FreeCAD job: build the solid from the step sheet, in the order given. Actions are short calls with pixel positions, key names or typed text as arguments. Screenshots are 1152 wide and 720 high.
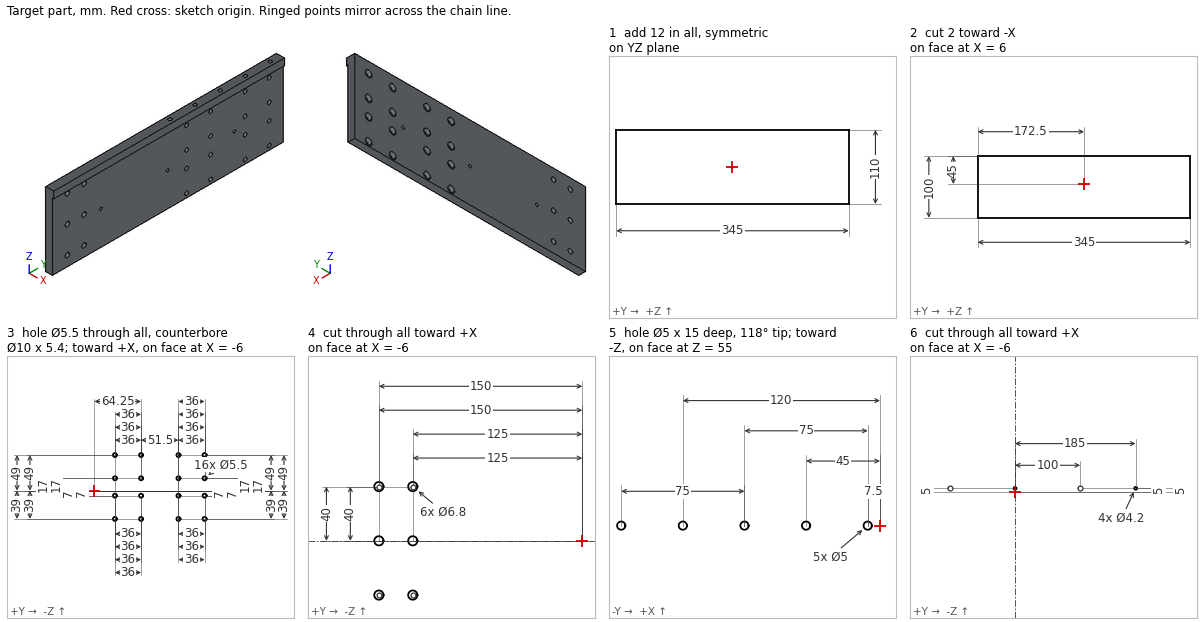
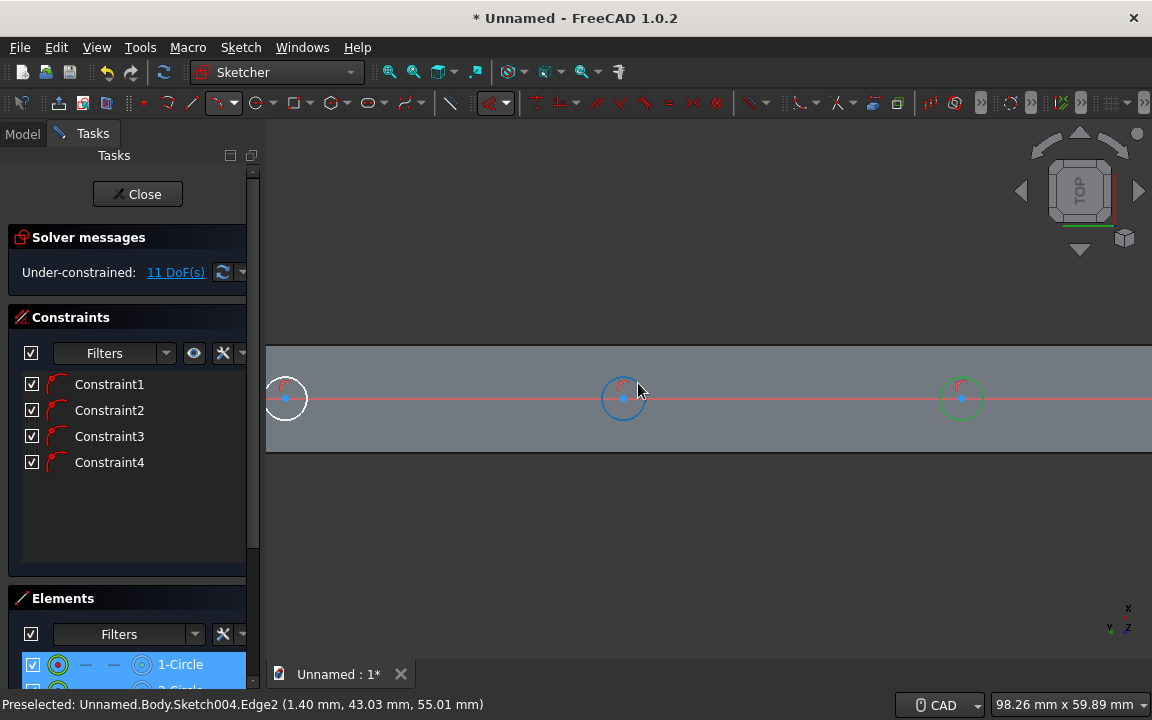
click(639, 383)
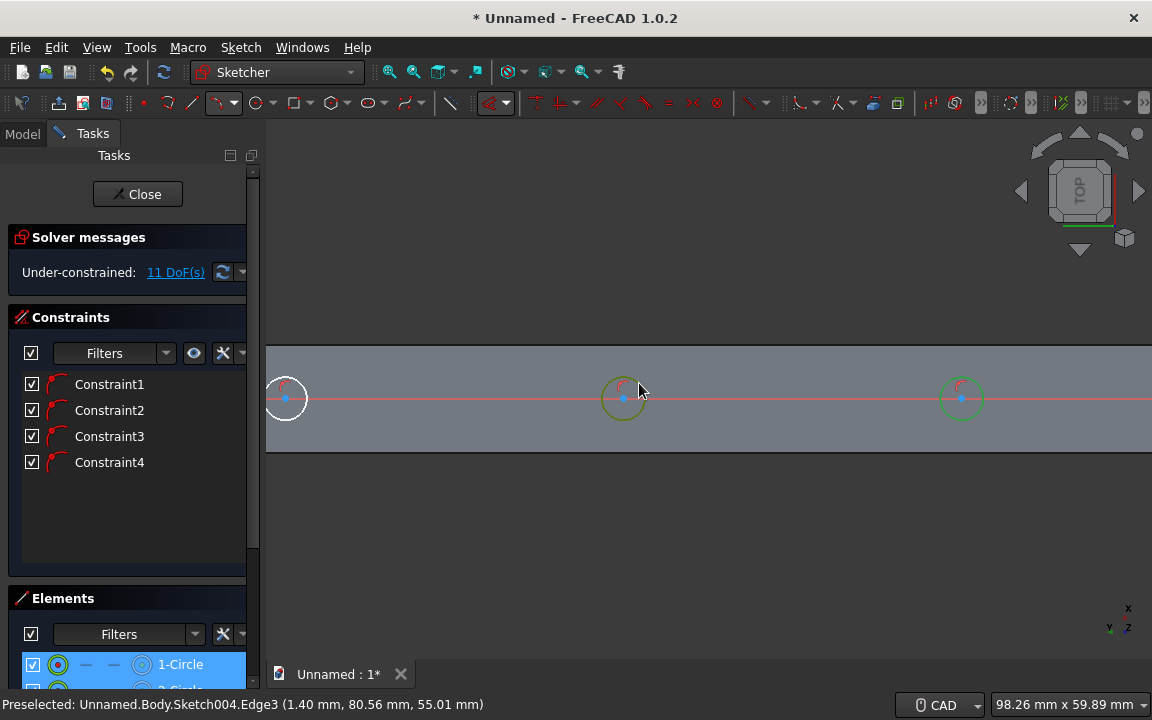
click(300, 383)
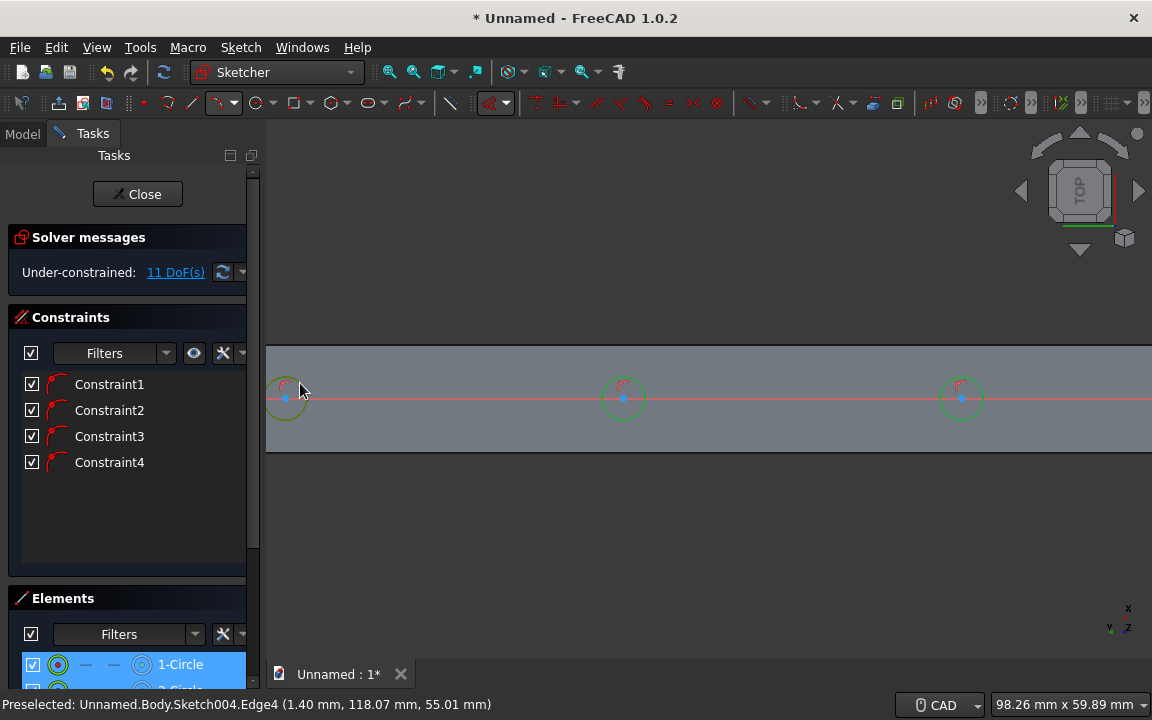
scroll(637, 383, down, 5)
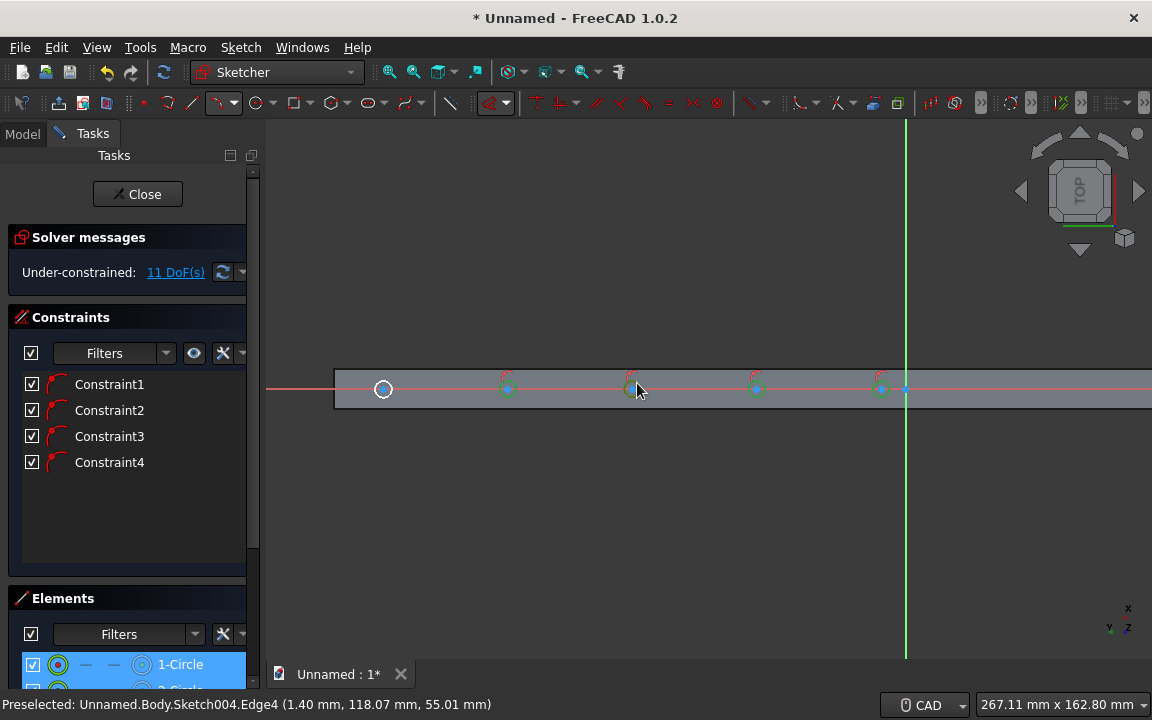
scroll(389, 383, up, 5)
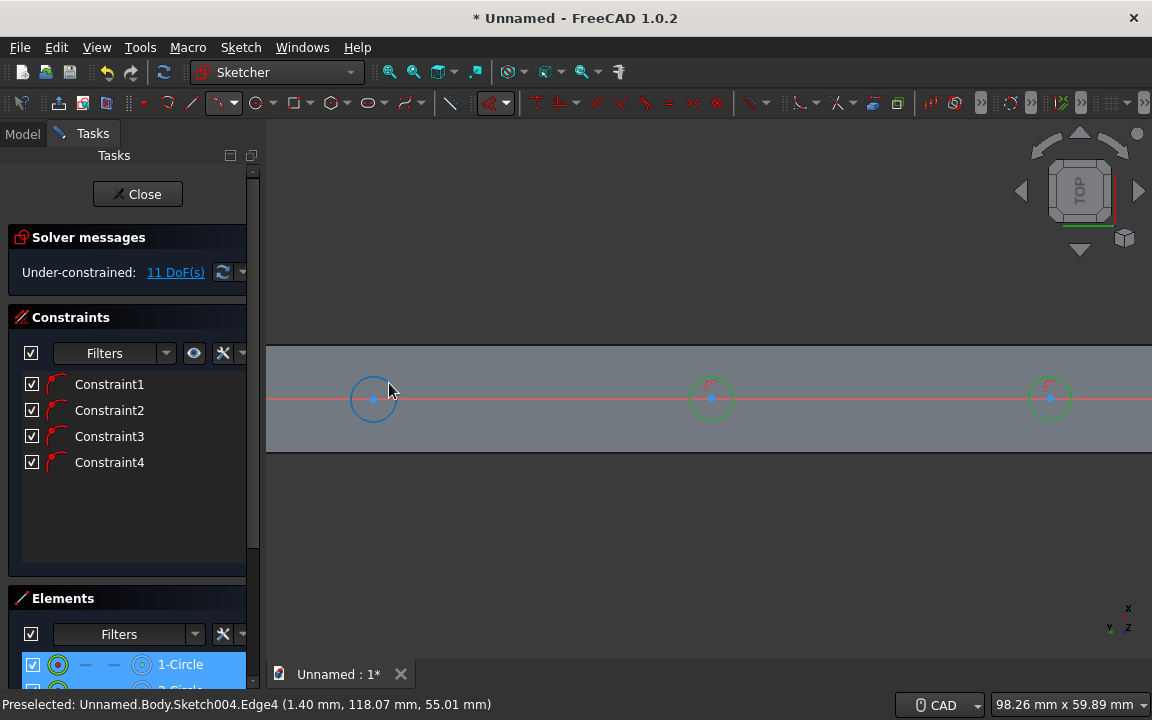
click(389, 383)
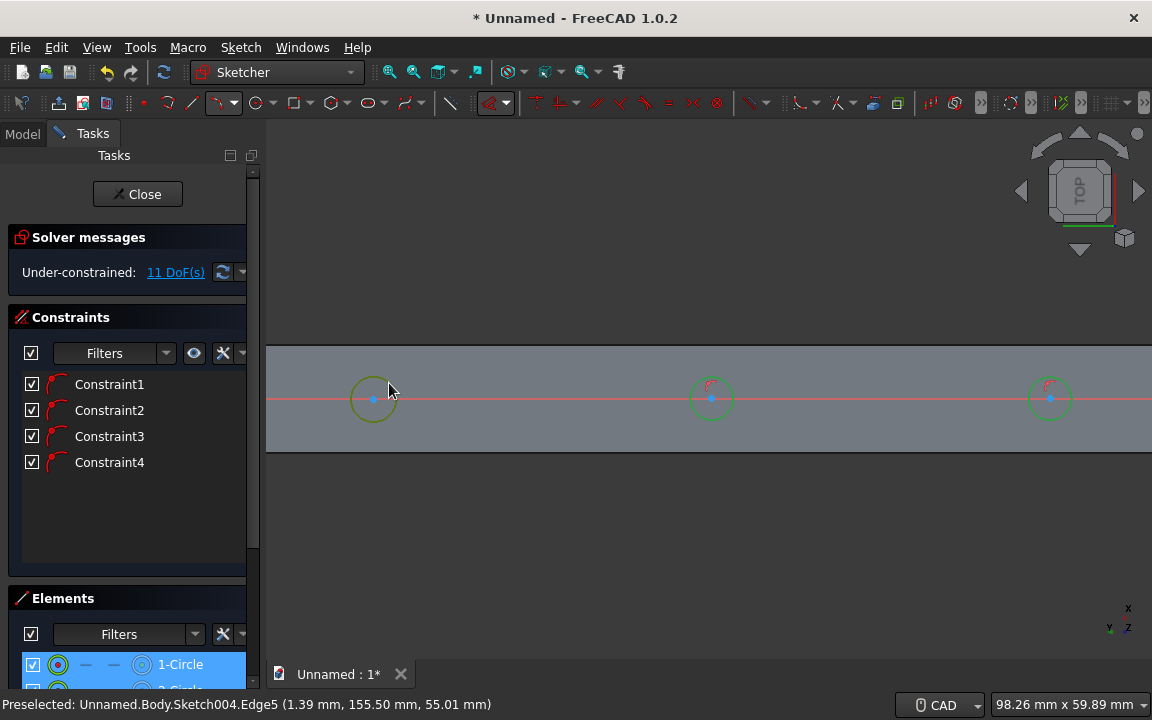
click(670, 104)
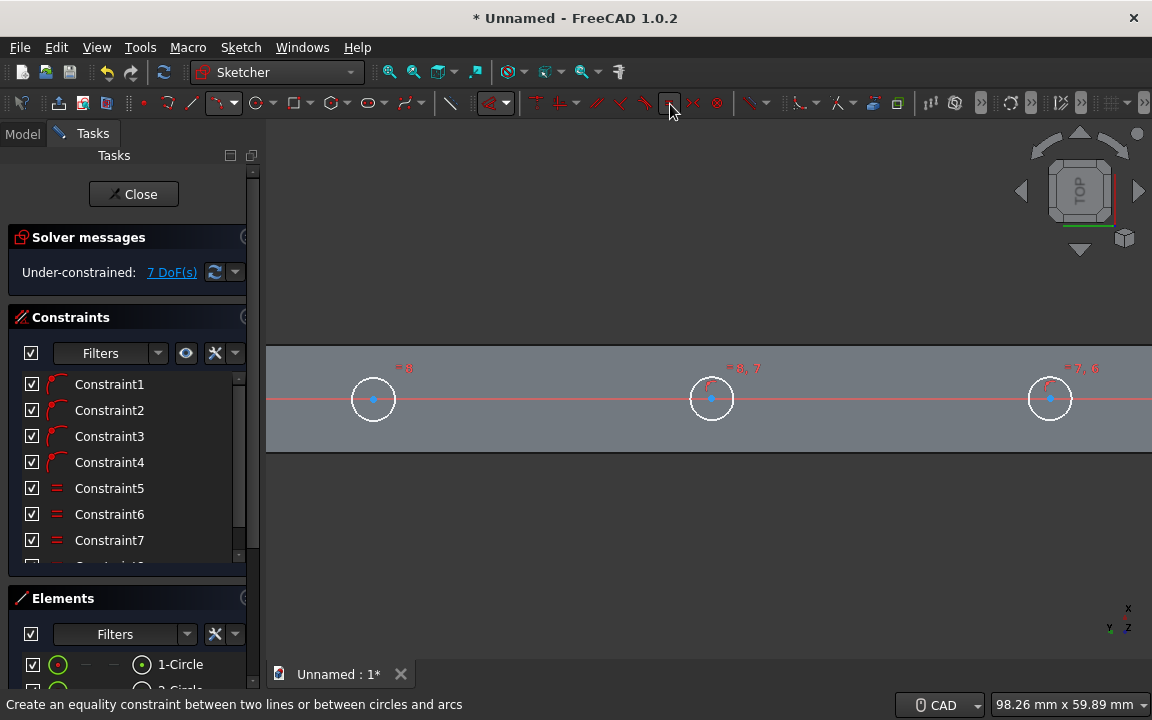
click(374, 399)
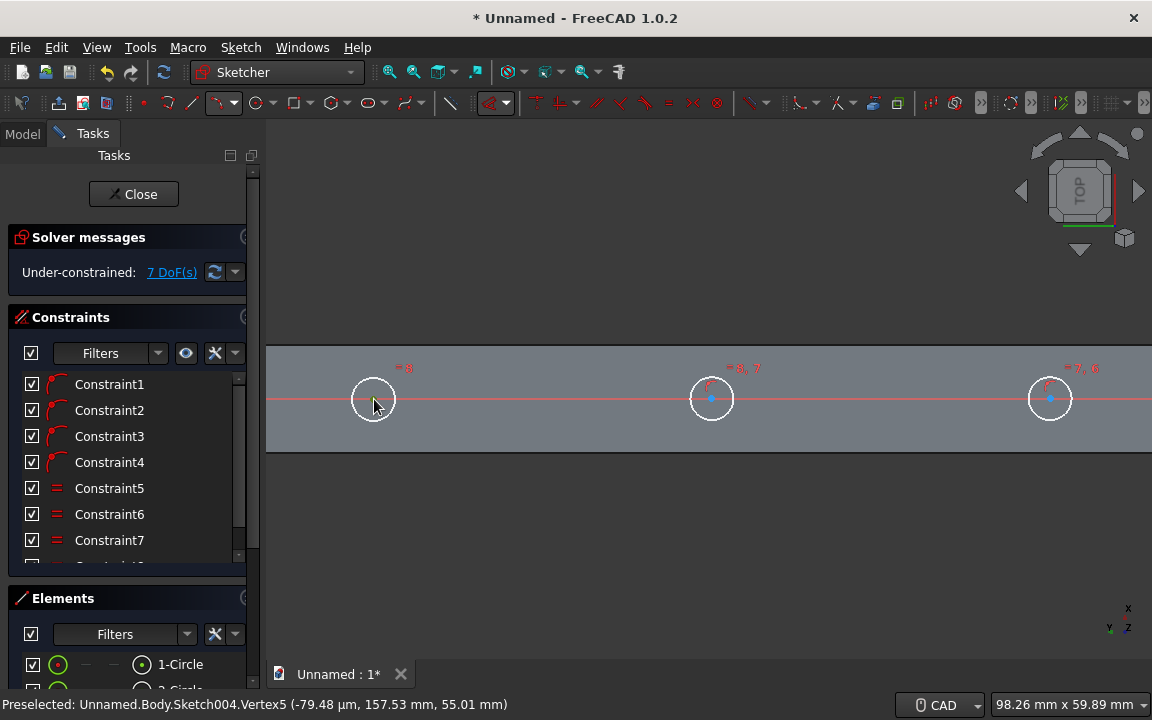
click(443, 399)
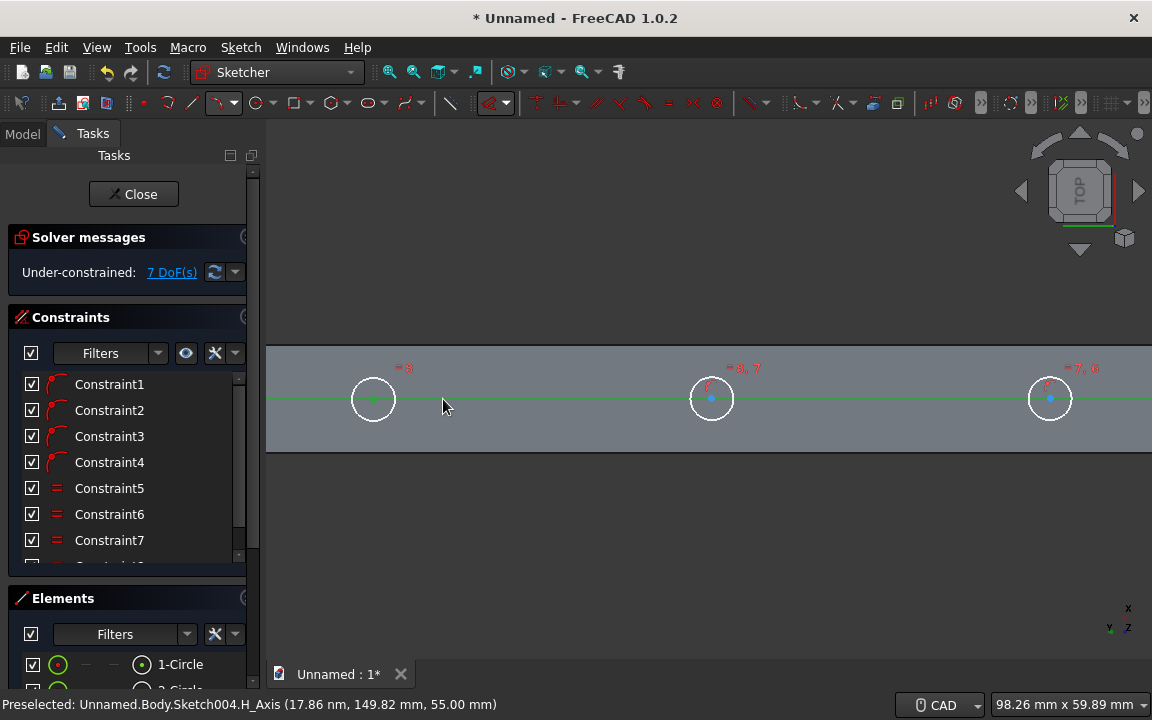
click(536, 104)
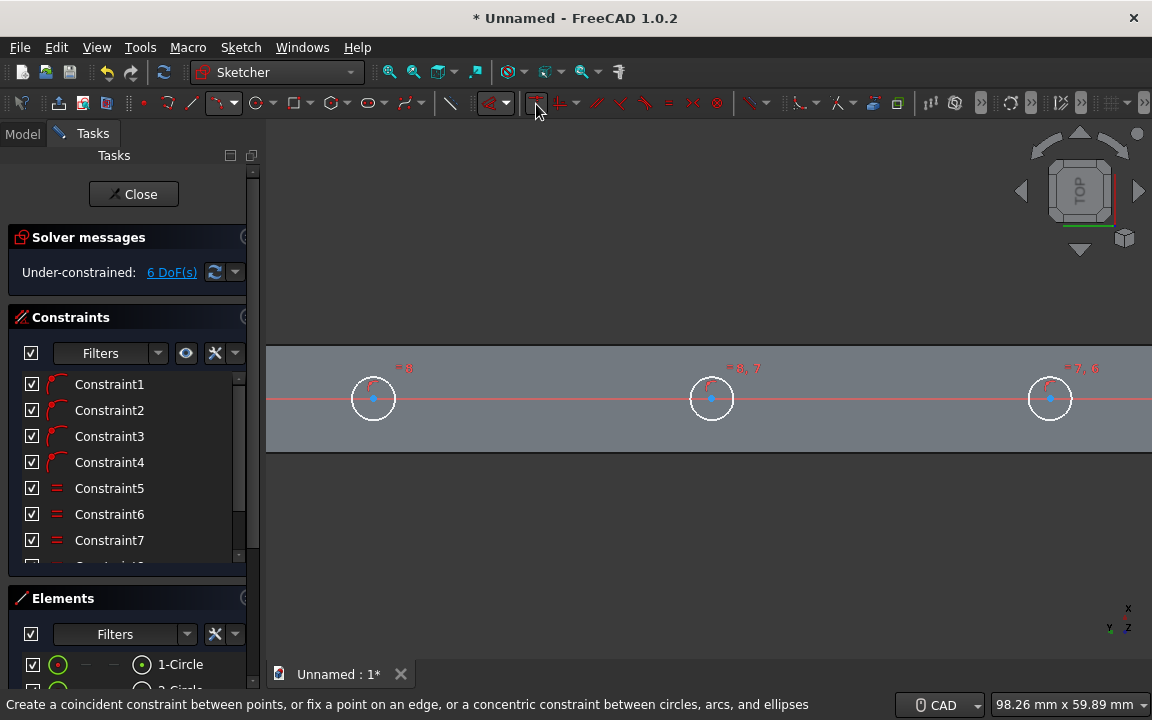
scroll(389, 383, down, 5)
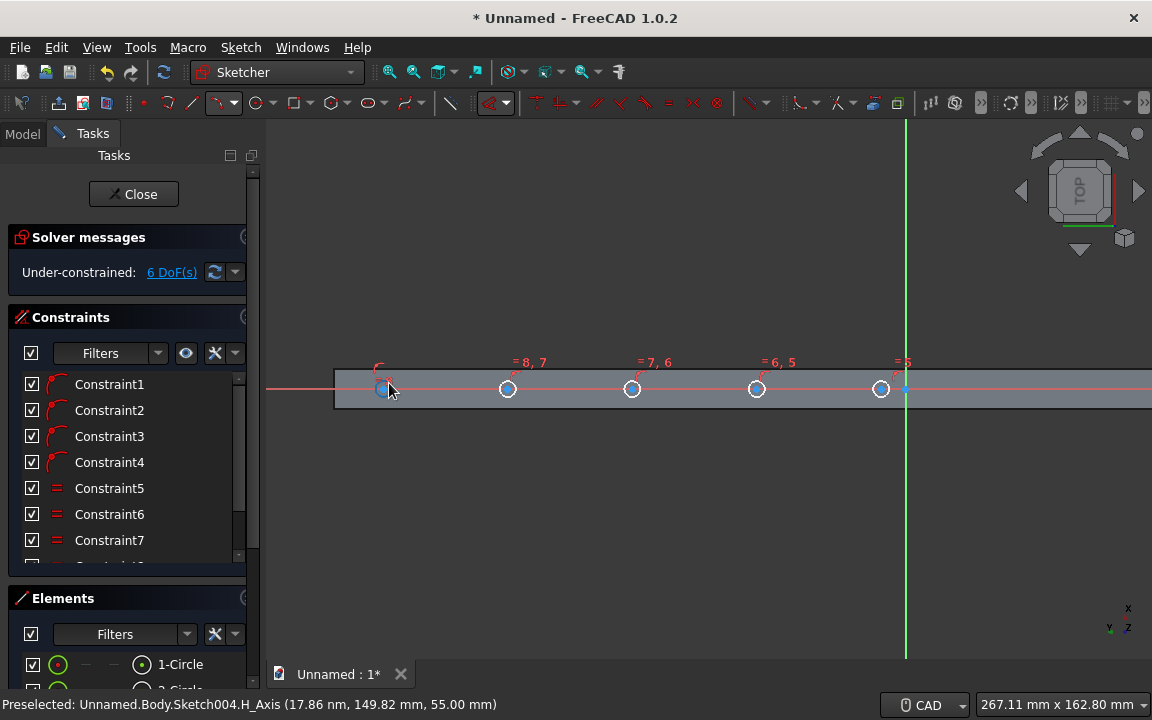
scroll(887, 383, up, 5)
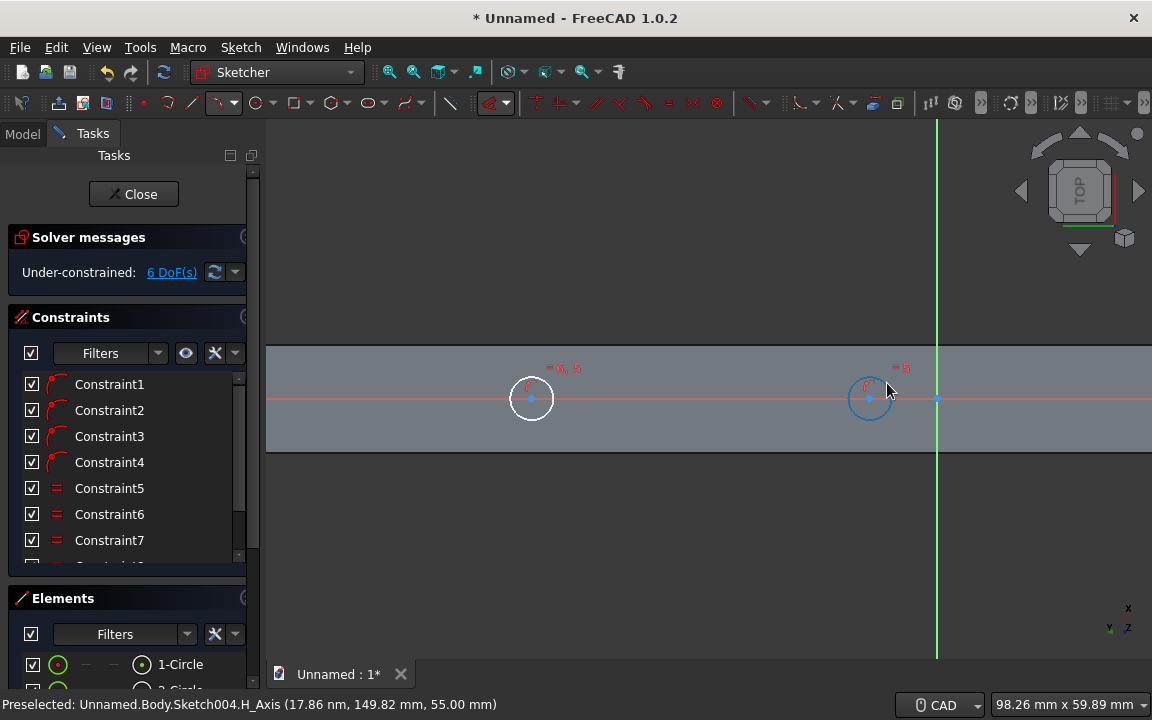
click(885, 383)